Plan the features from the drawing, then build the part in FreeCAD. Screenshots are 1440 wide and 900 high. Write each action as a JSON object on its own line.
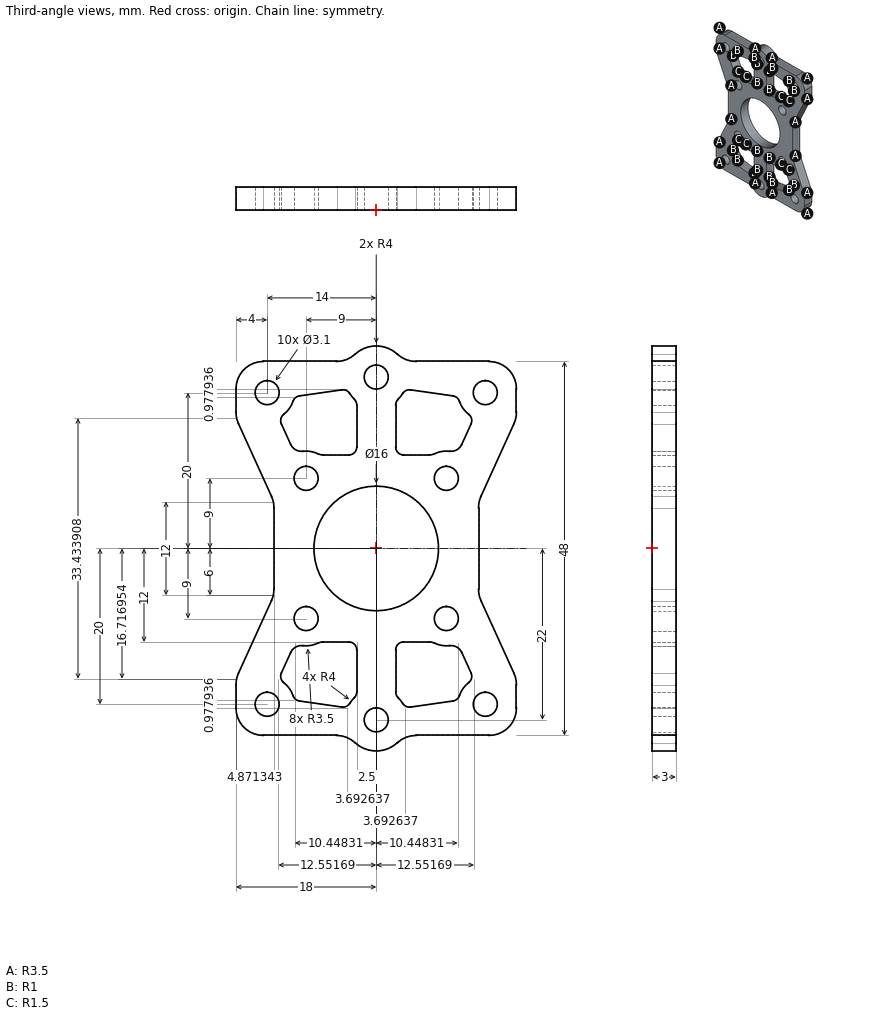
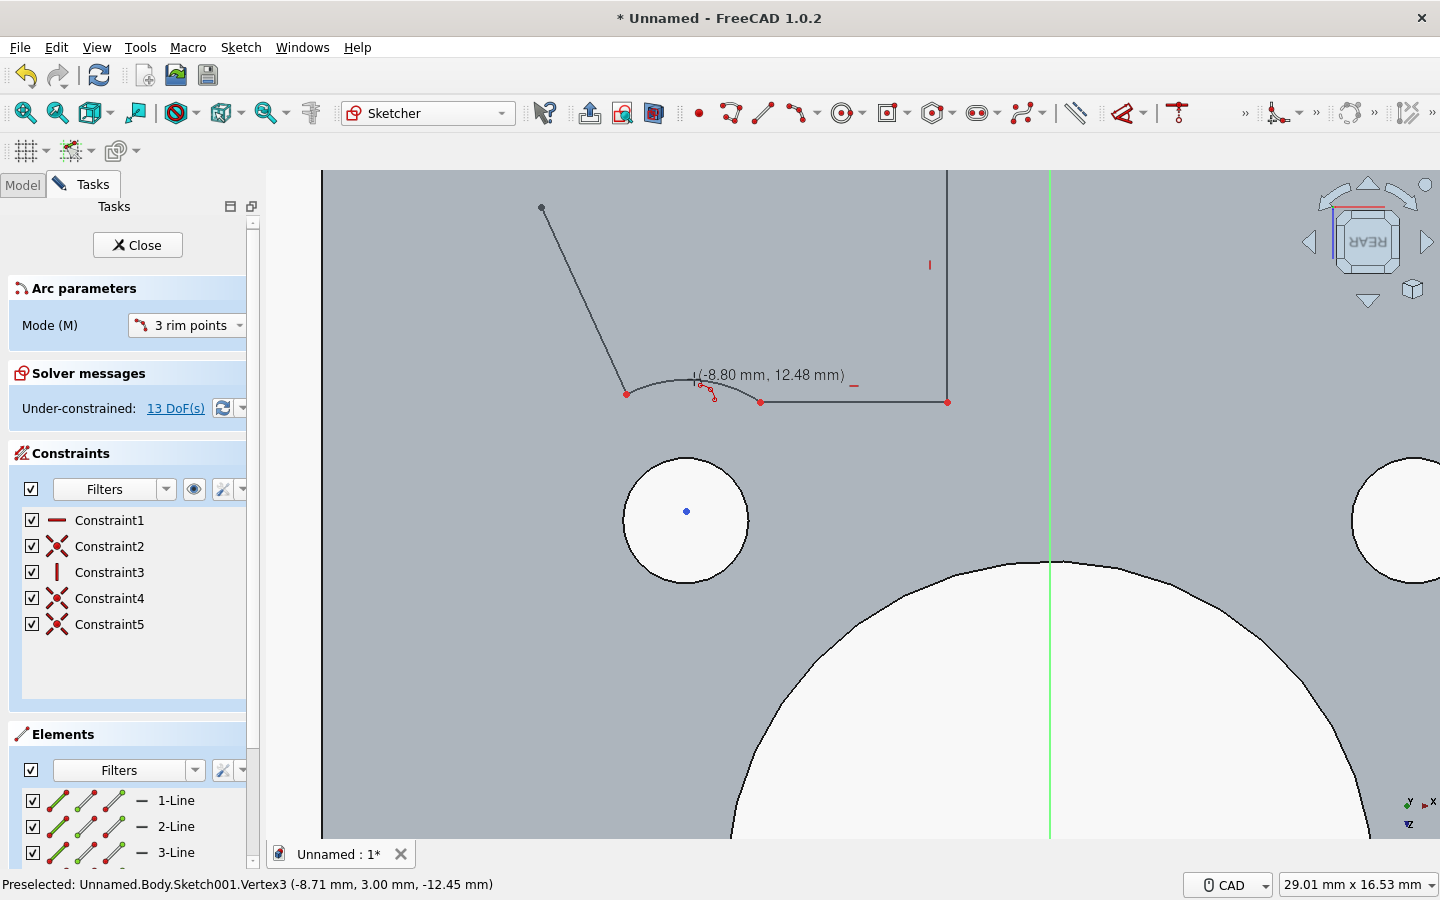
{"action": "scroll", "coordinate": [698, 380], "scroll_direction": "down", "scroll_amount": 7}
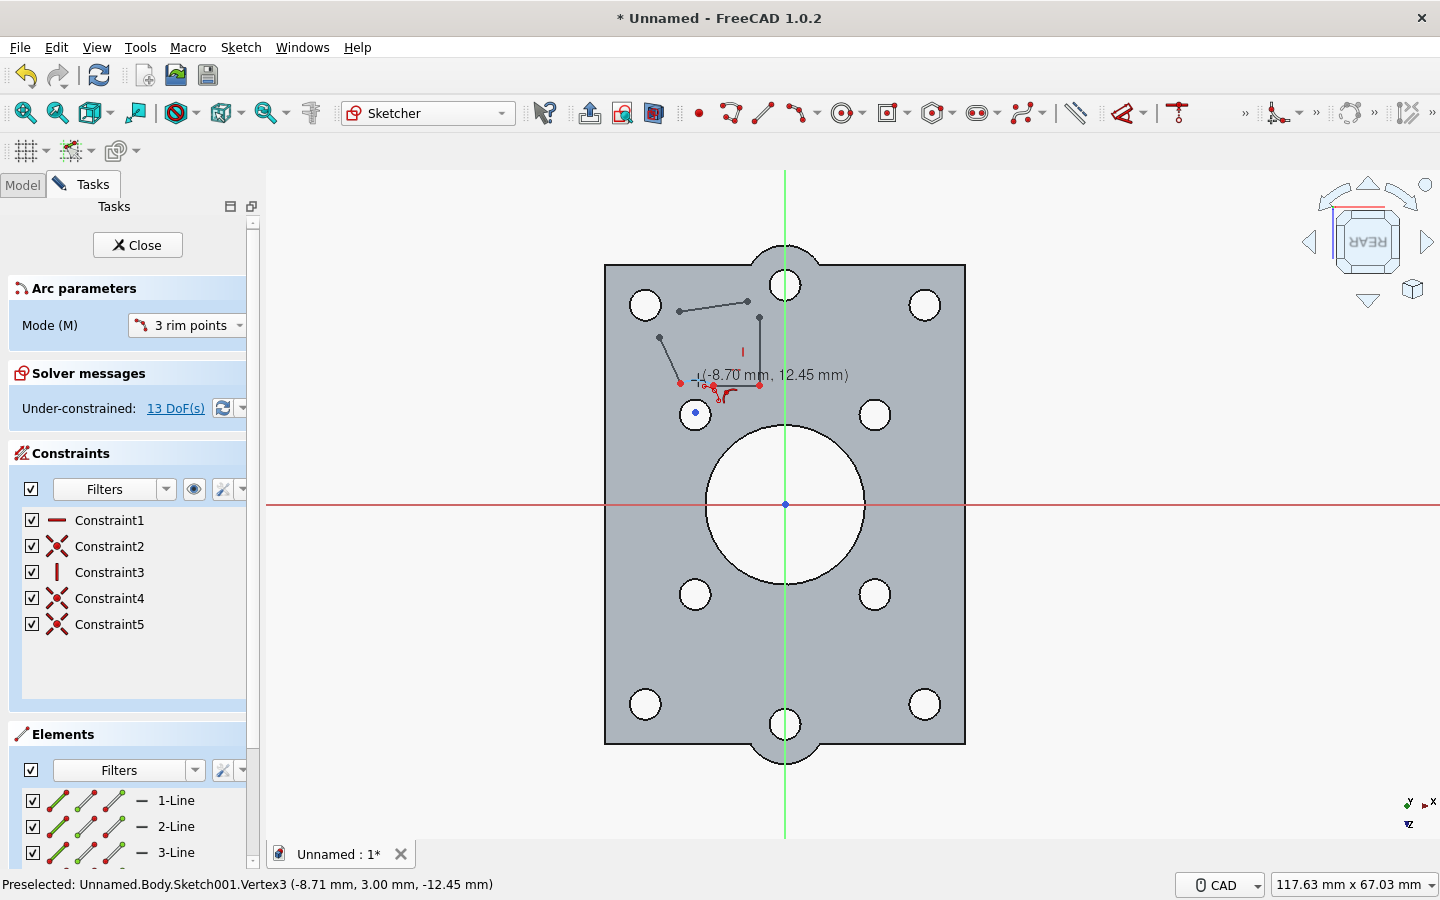
{"action": "left_click", "coordinate": [760, 318]}
{"action": "left_click", "coordinate": [748, 302]}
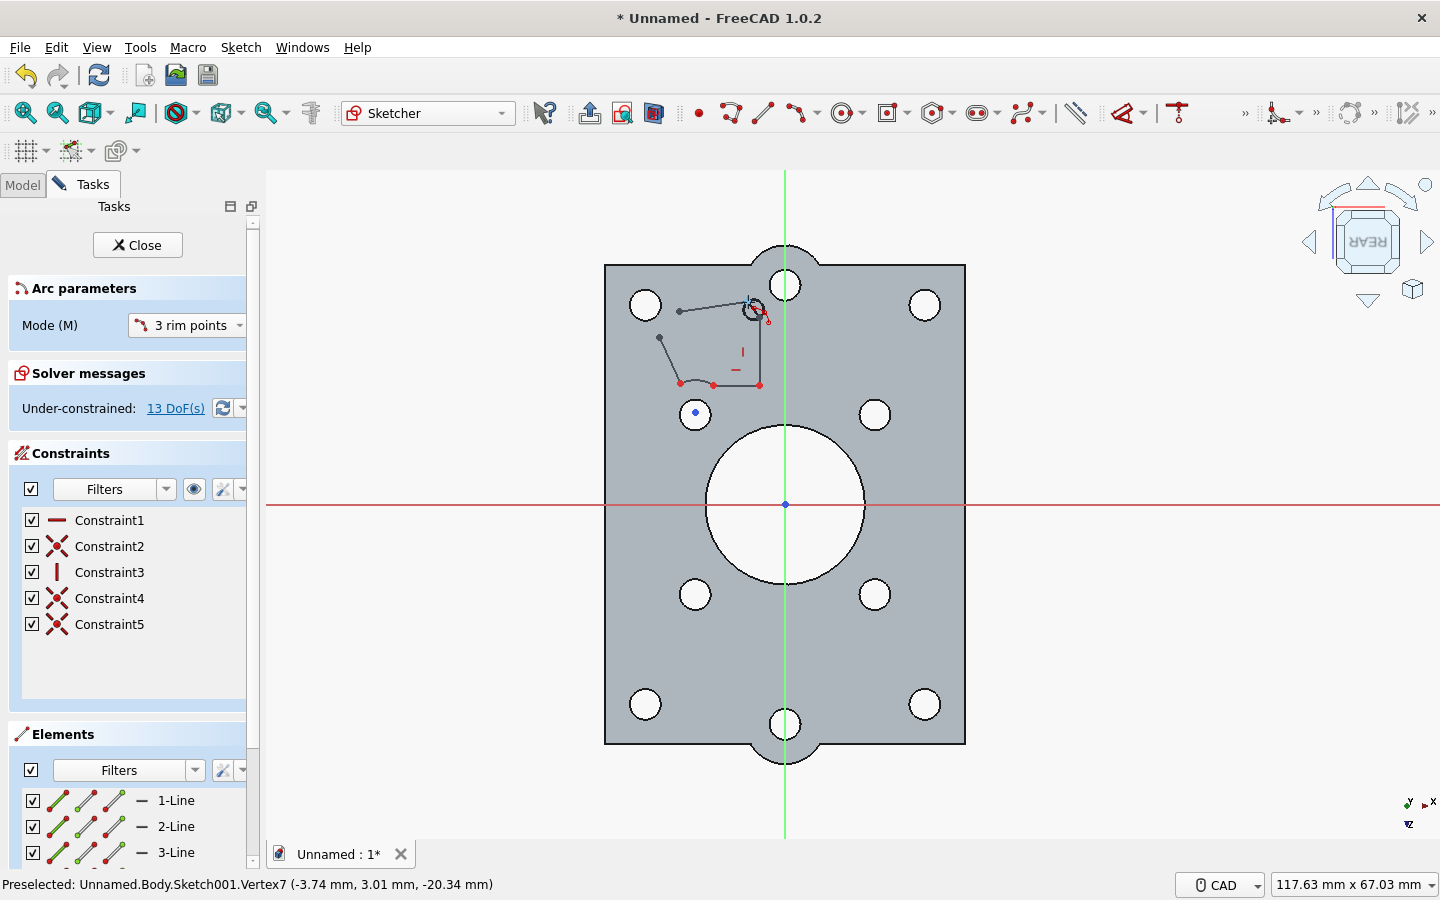
{"action": "scroll", "coordinate": [753, 309], "scroll_direction": "up", "scroll_amount": 13}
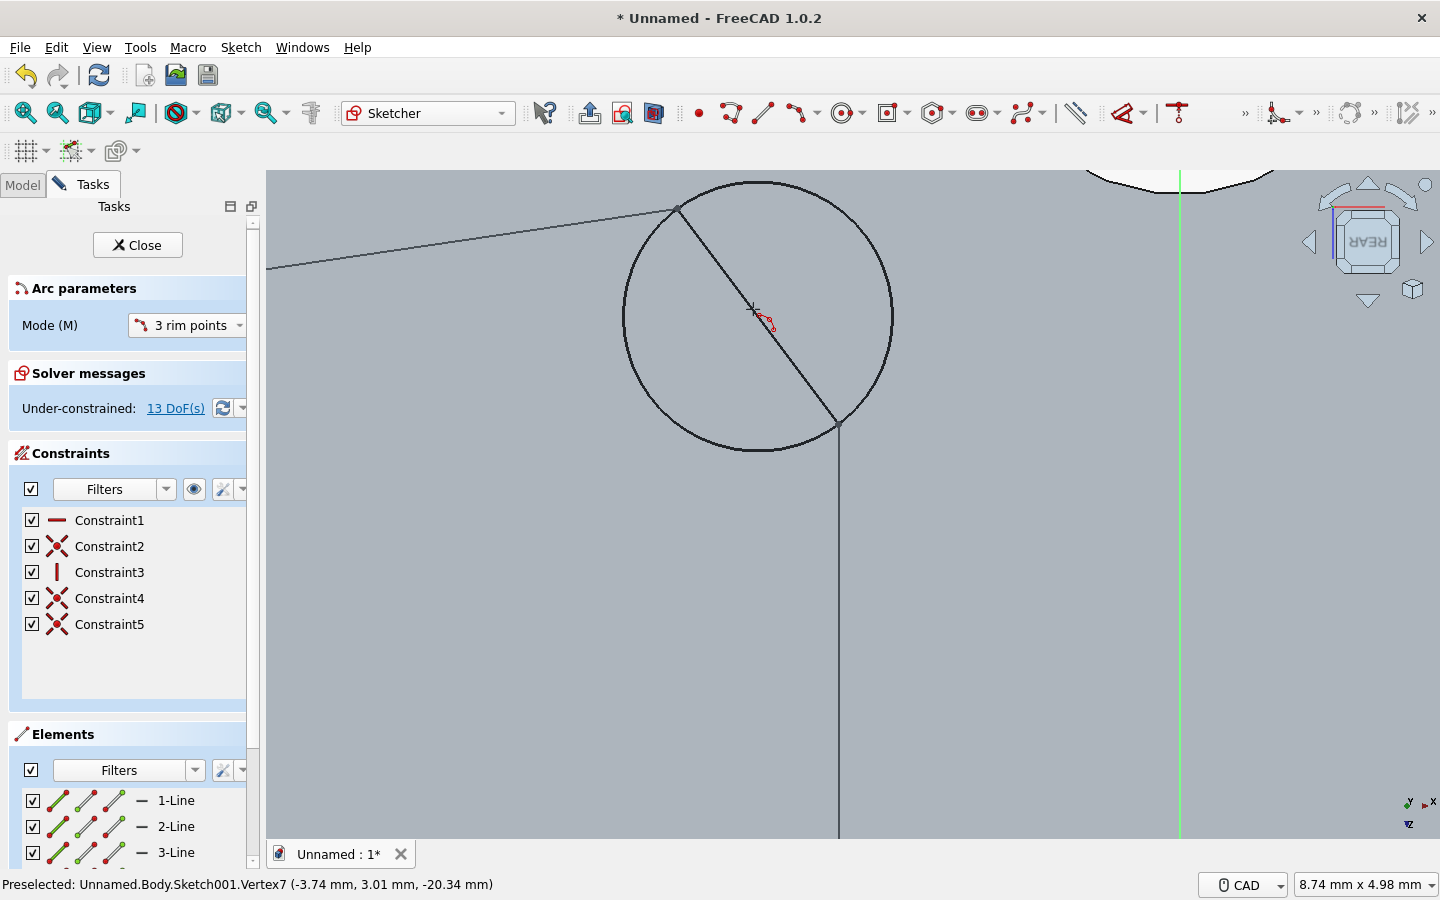
{"action": "left_click", "coordinate": [750, 309]}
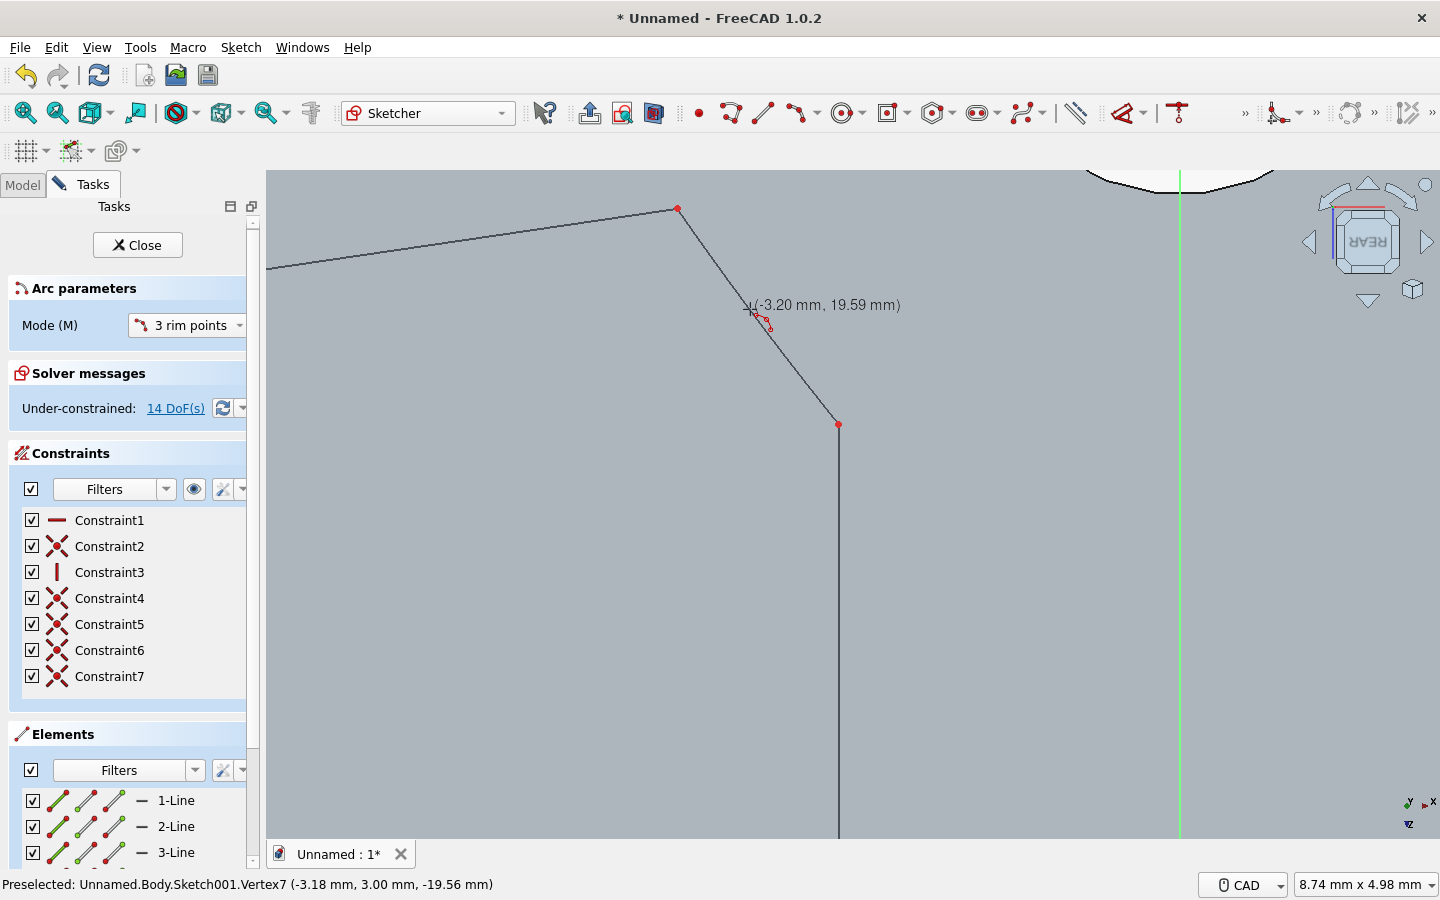
{"action": "scroll", "coordinate": [753, 309], "scroll_direction": "down", "scroll_amount": 13}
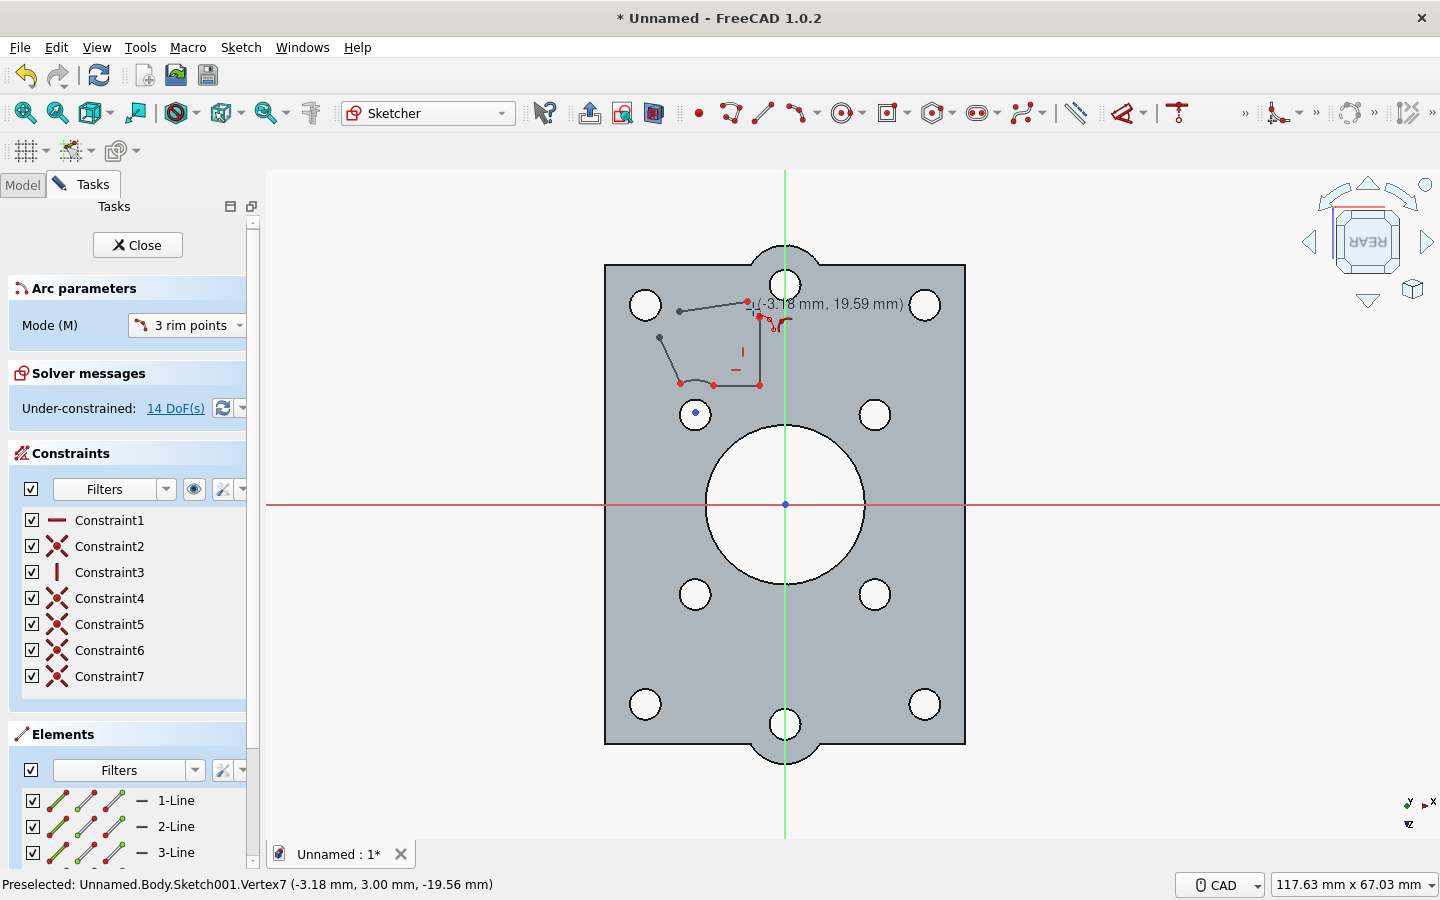
{"action": "left_click", "coordinate": [680, 312]}
{"action": "left_click", "coordinate": [660, 338]}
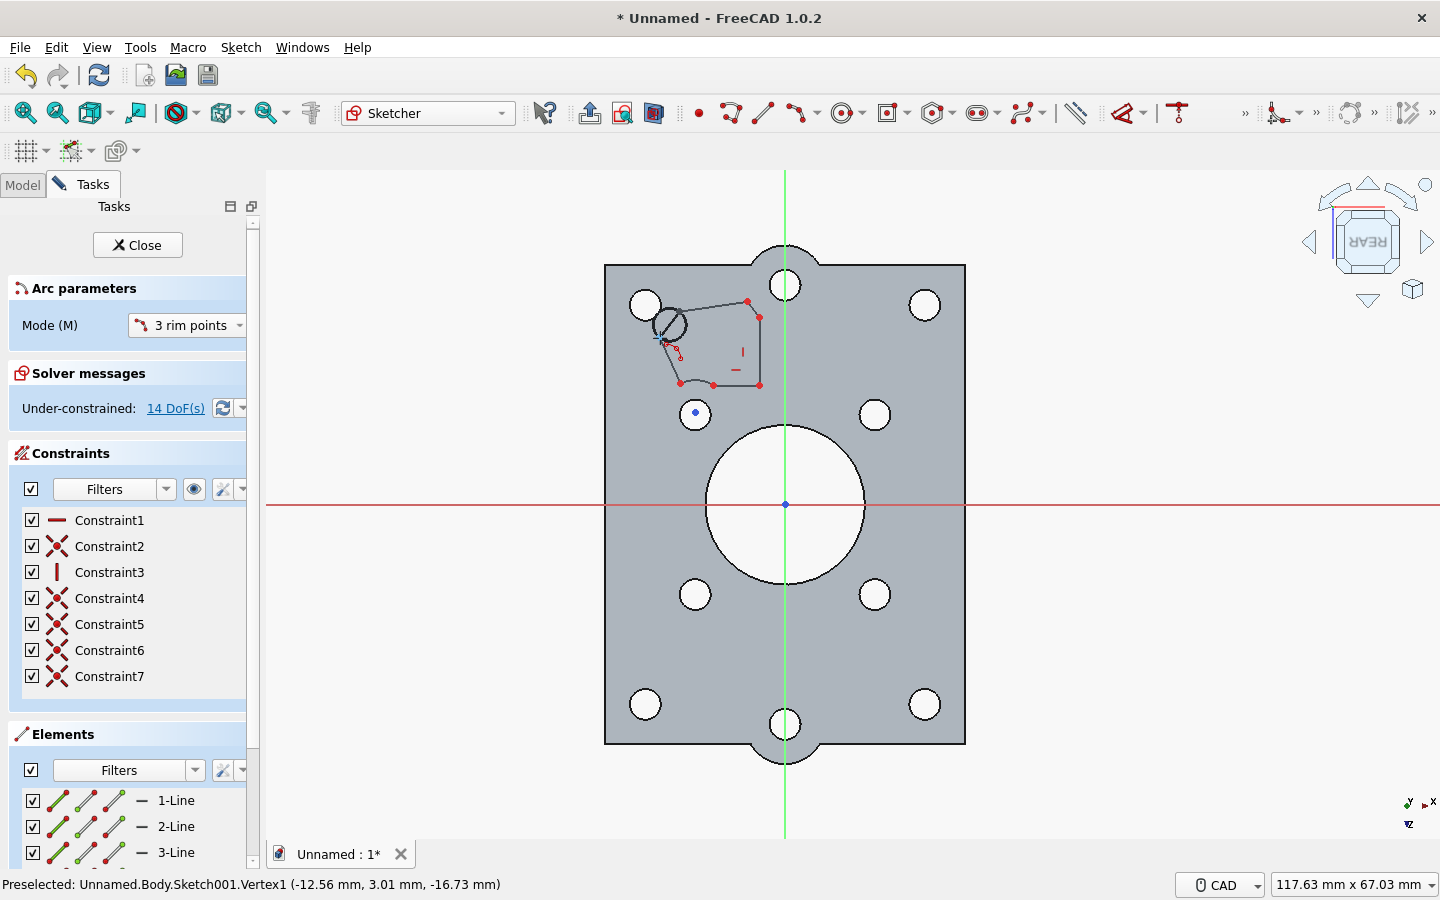
{"action": "scroll", "coordinate": [673, 326], "scroll_direction": "up", "scroll_amount": 7}